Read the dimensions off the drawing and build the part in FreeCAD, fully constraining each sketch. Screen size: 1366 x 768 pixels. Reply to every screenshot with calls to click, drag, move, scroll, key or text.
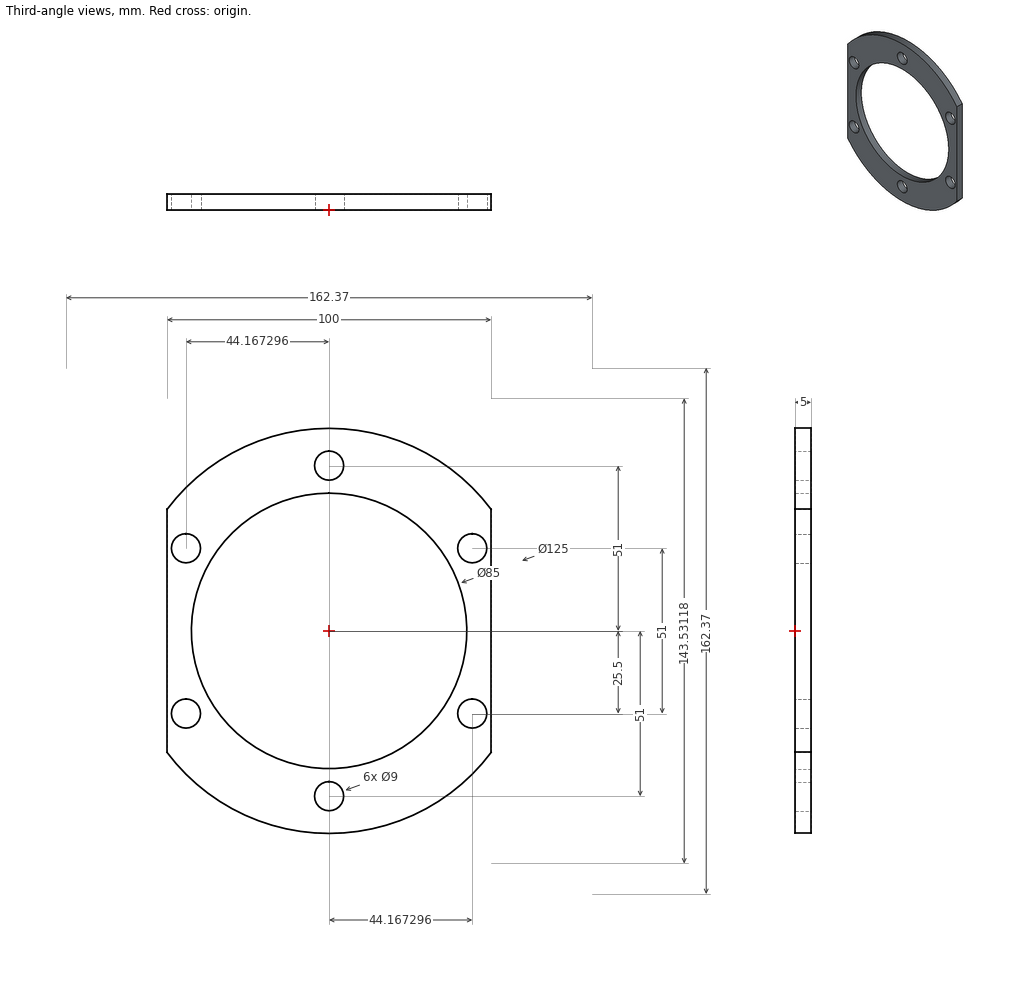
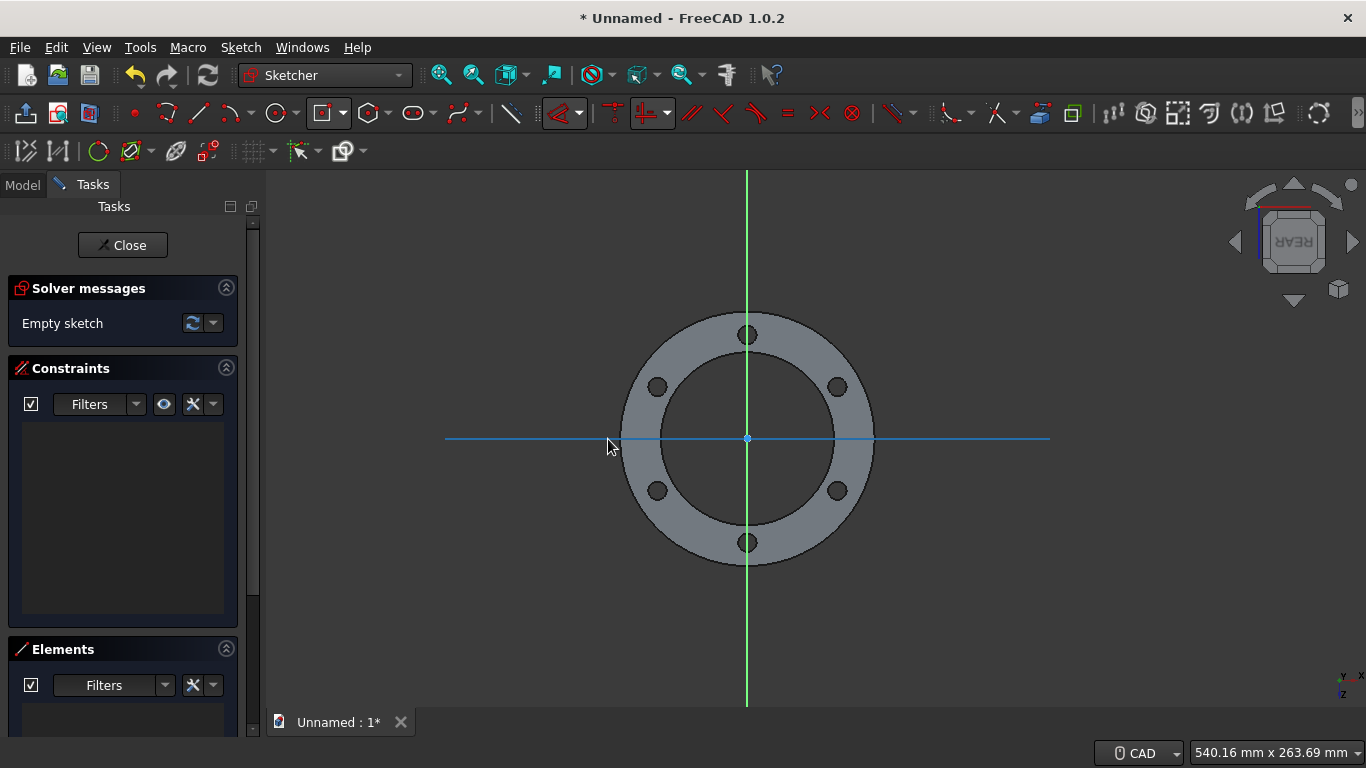
click(322, 114)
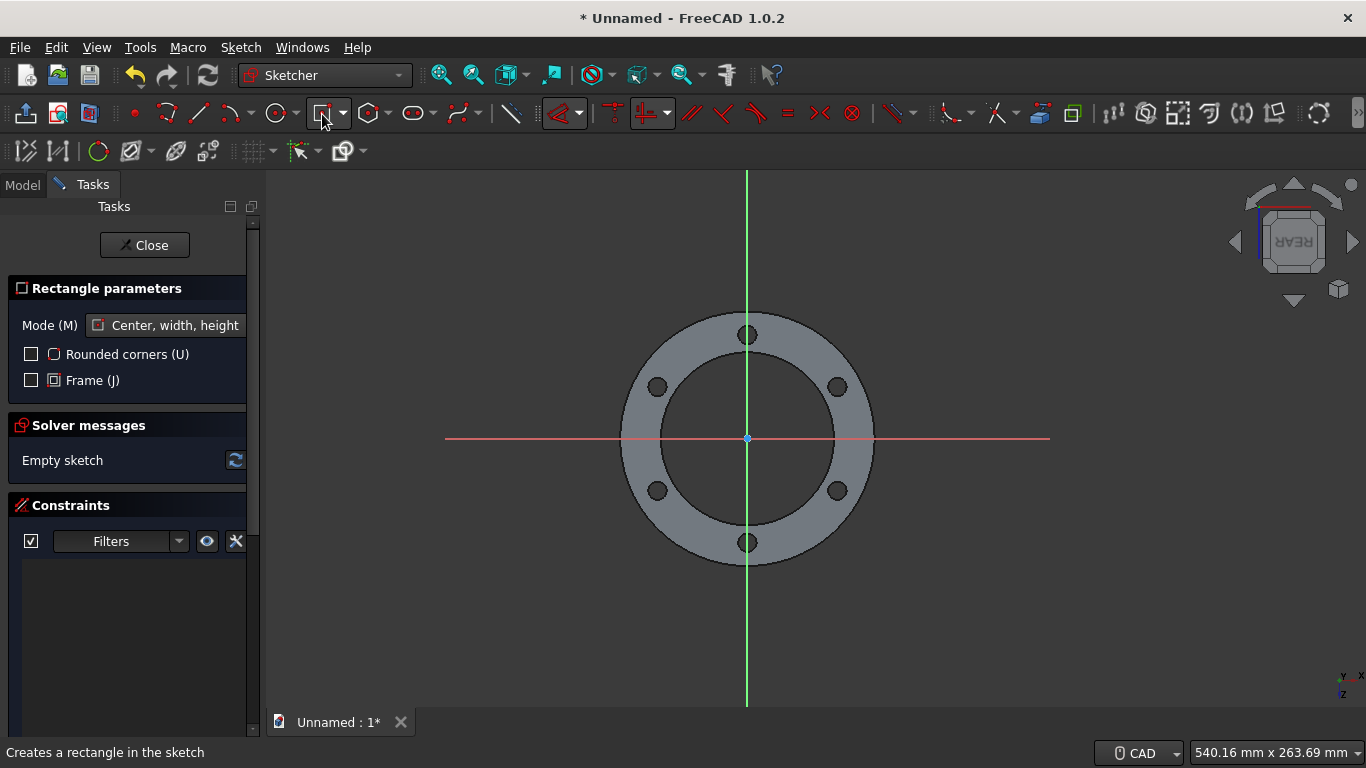
click(747, 439)
move(913, 274)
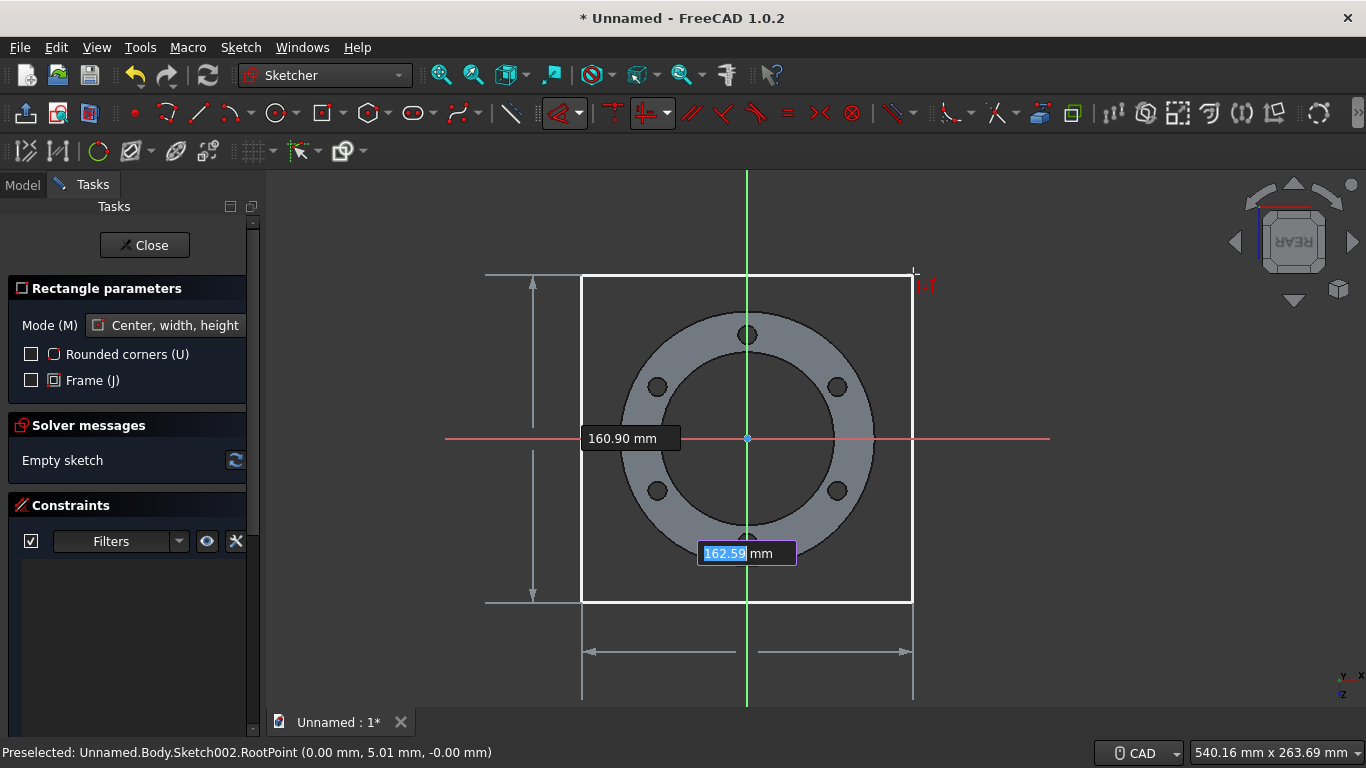
text(162.37)
key(Tab)
text(162.37)
key(Return)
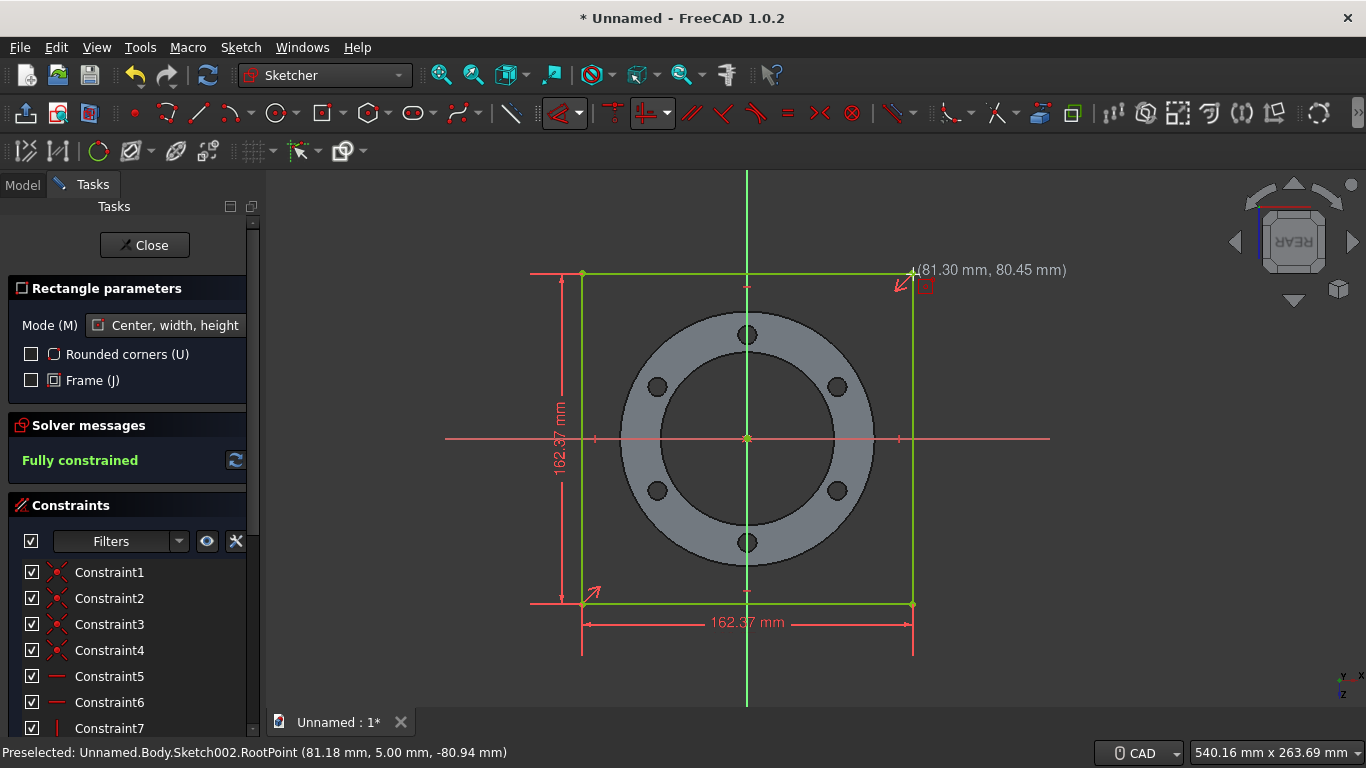
click(747, 439)
move(849, 293)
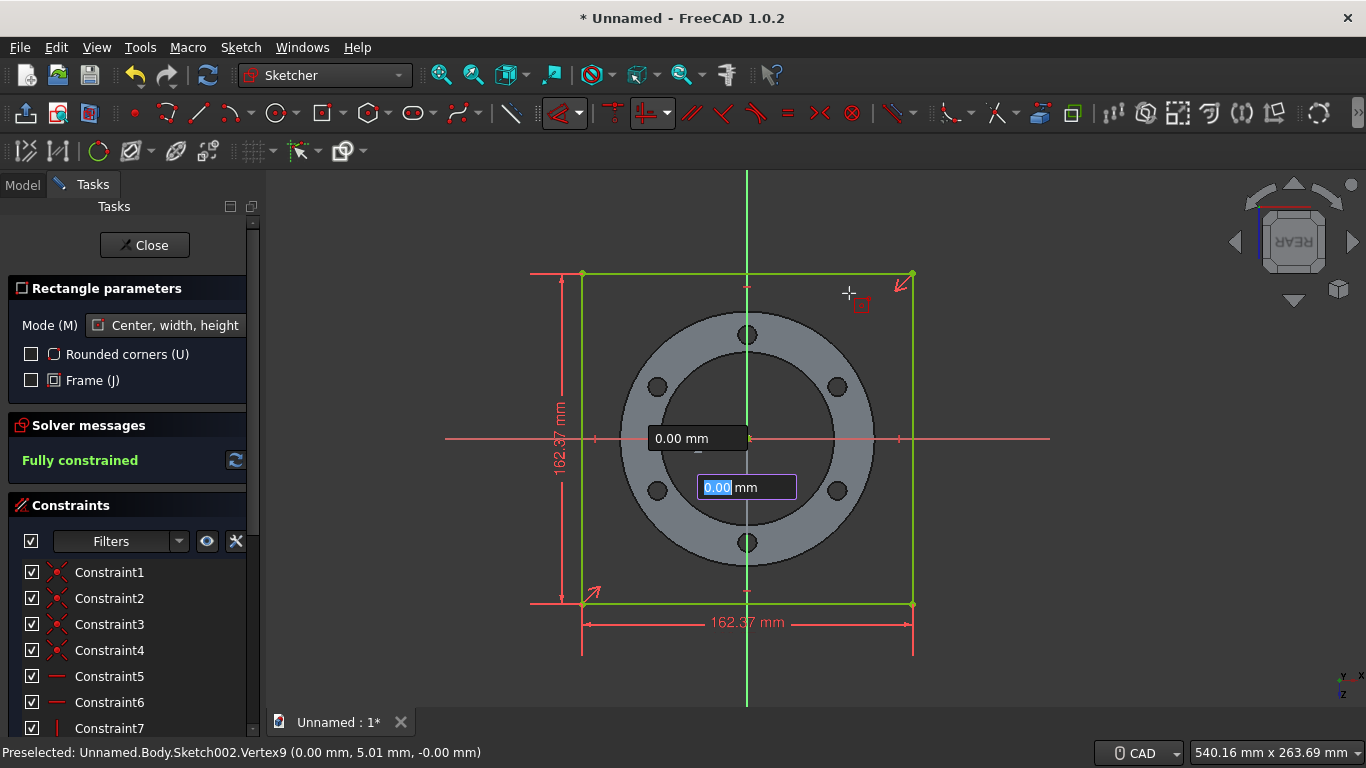
text(100)
key(Tab)
text(143.53118)
key(Return)
key(Escape)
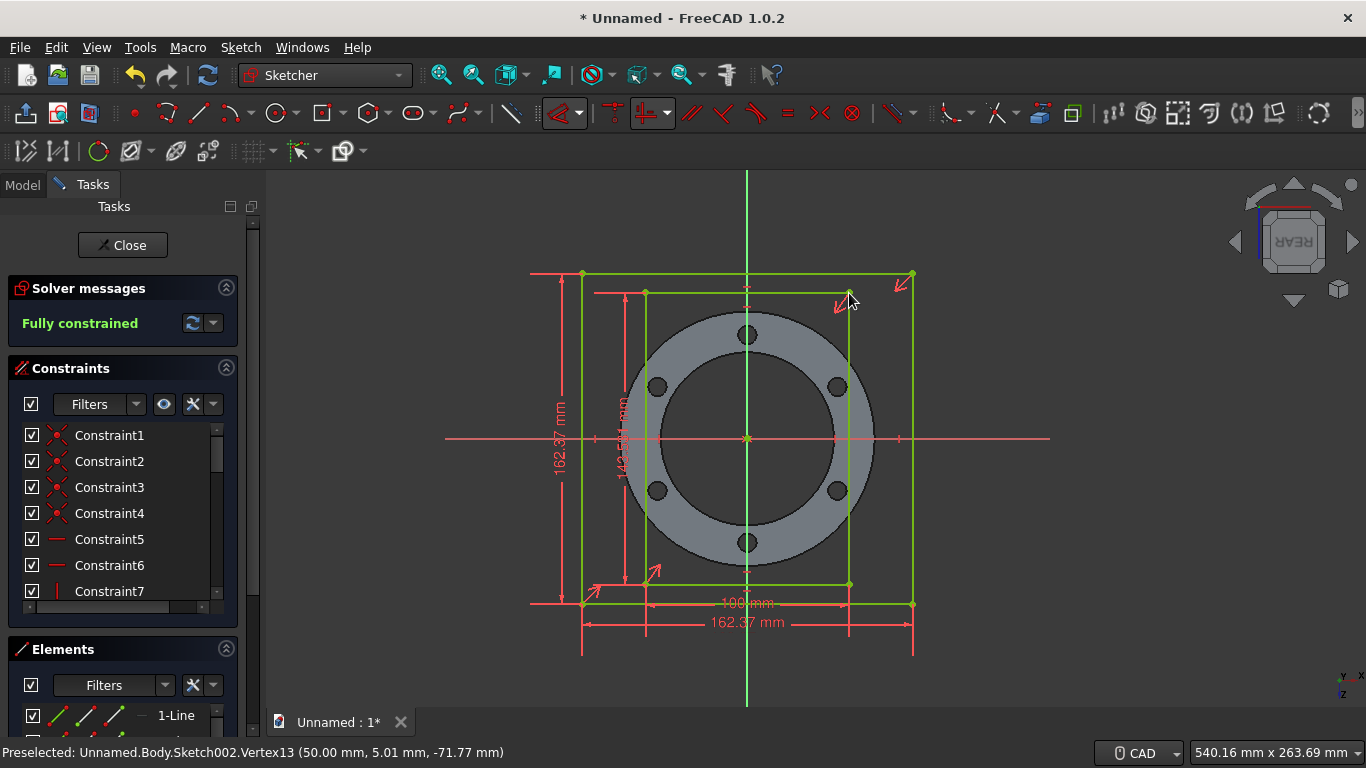
click(123, 245)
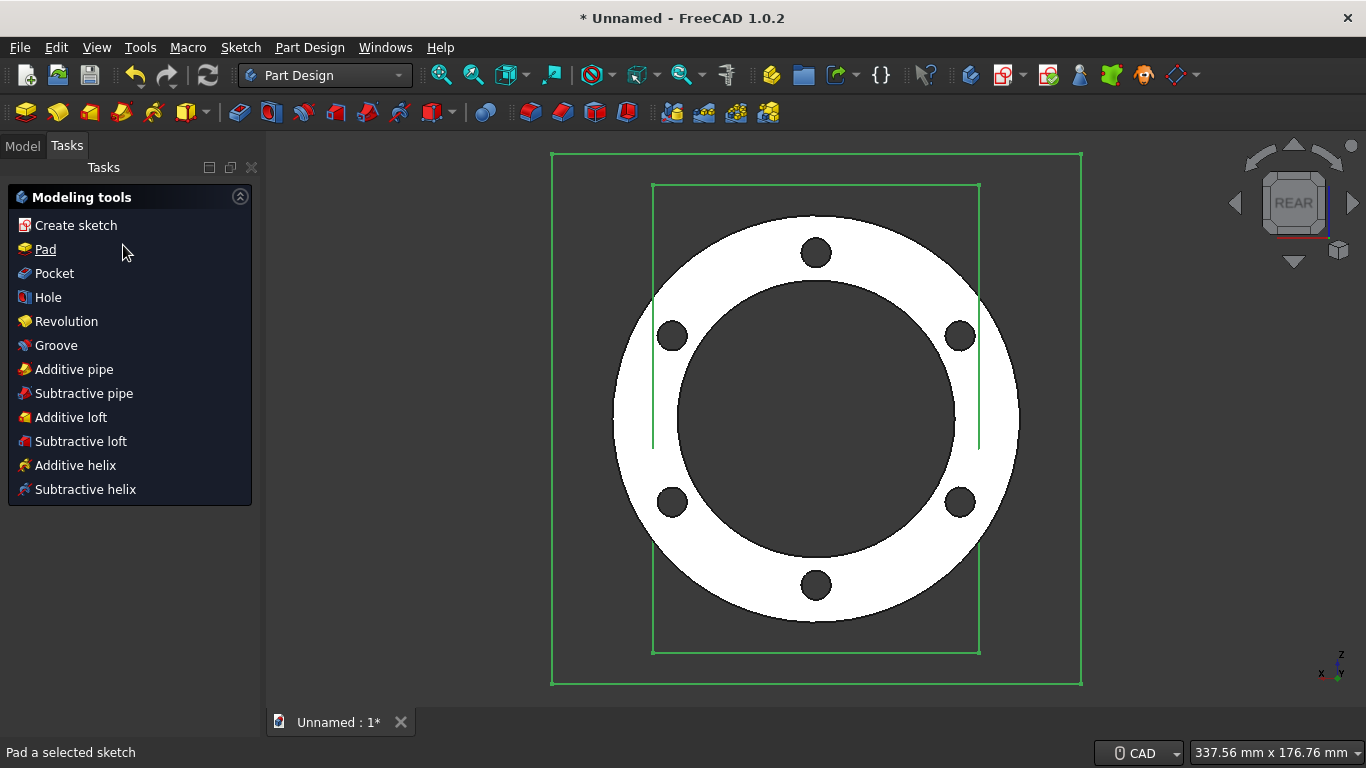
click(240, 112)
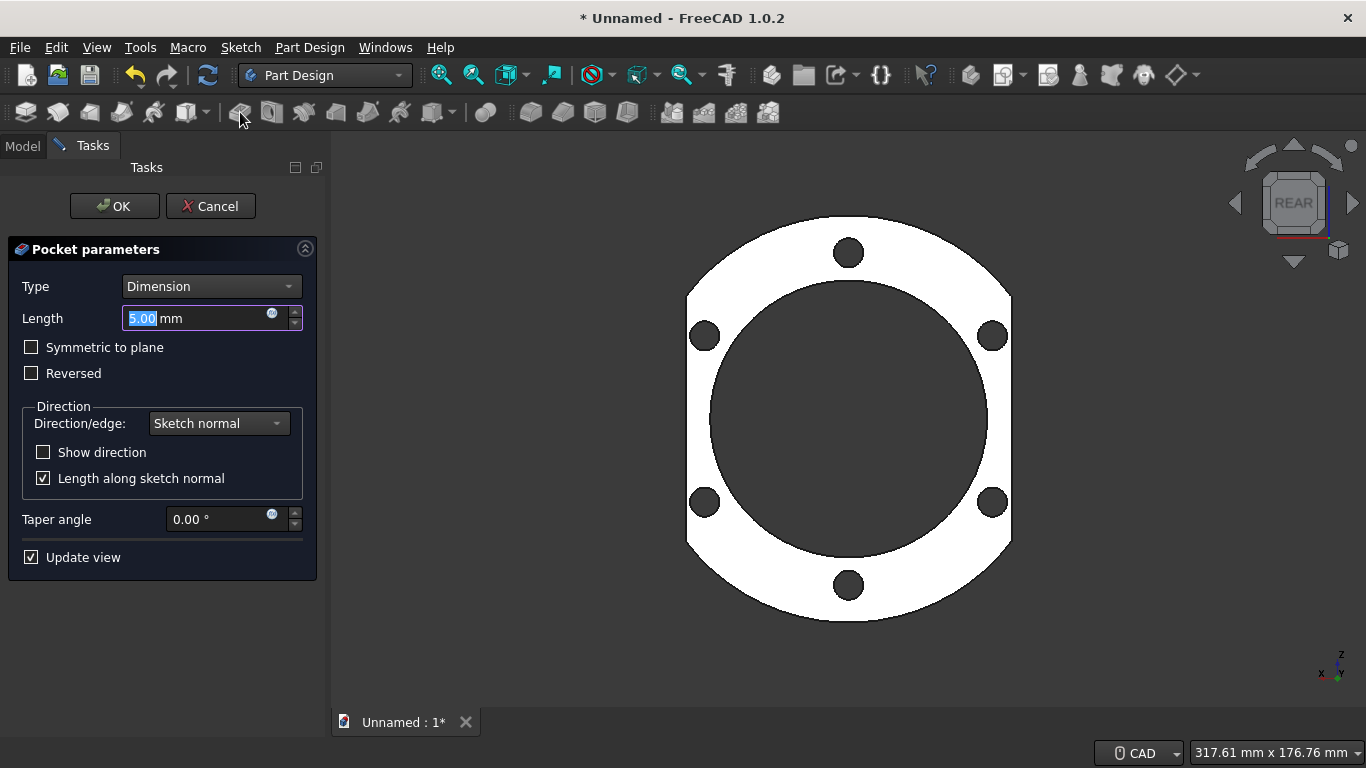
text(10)
key(Tab)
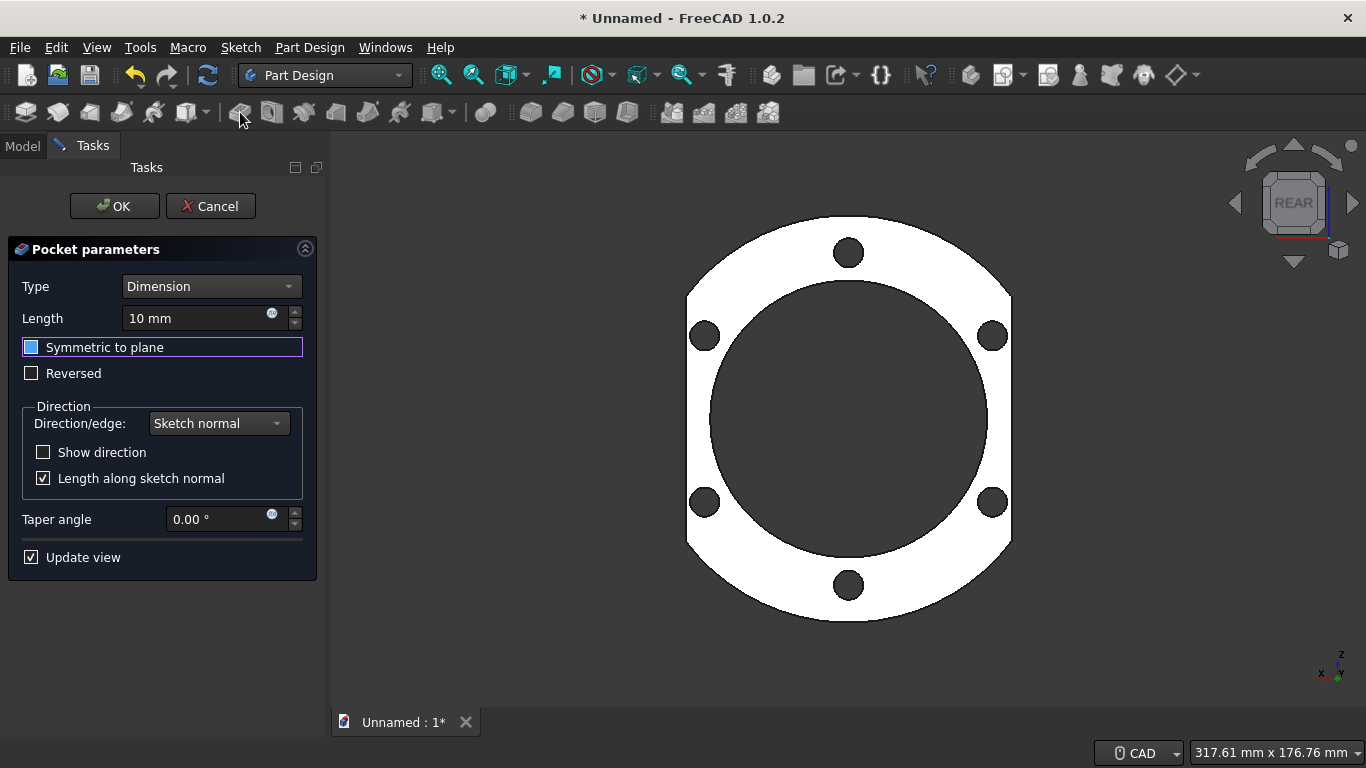
click(115, 206)